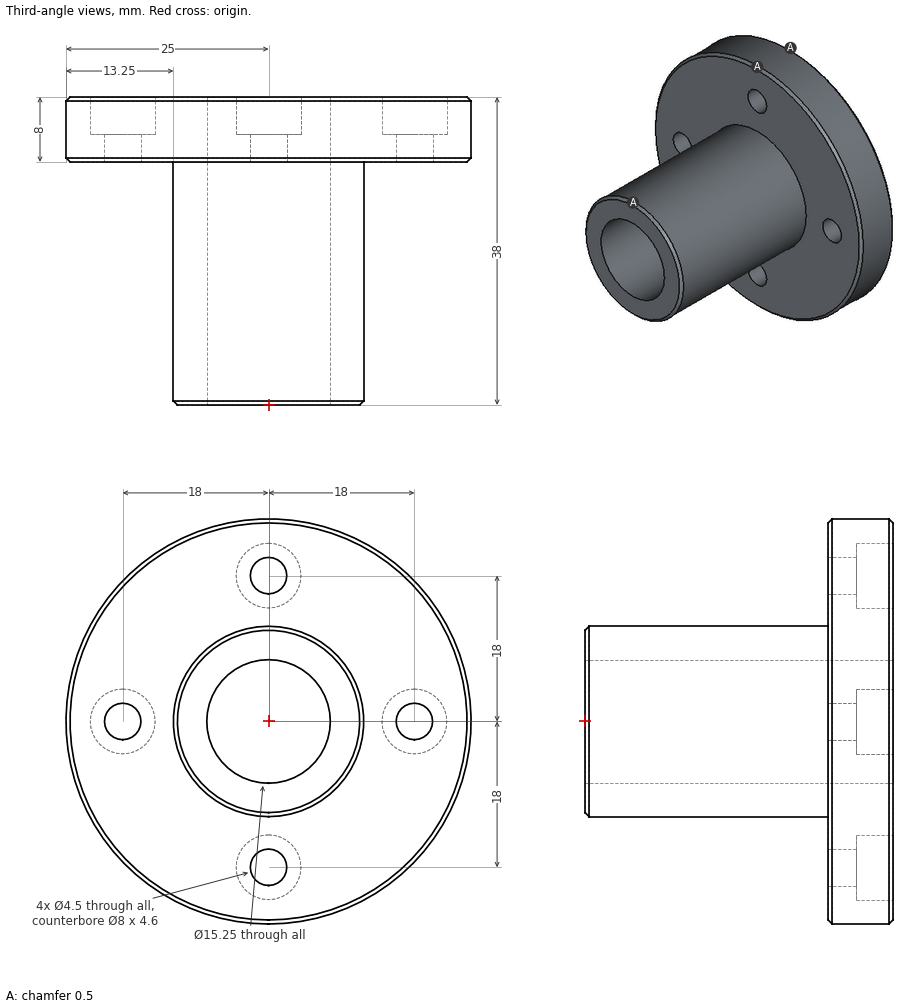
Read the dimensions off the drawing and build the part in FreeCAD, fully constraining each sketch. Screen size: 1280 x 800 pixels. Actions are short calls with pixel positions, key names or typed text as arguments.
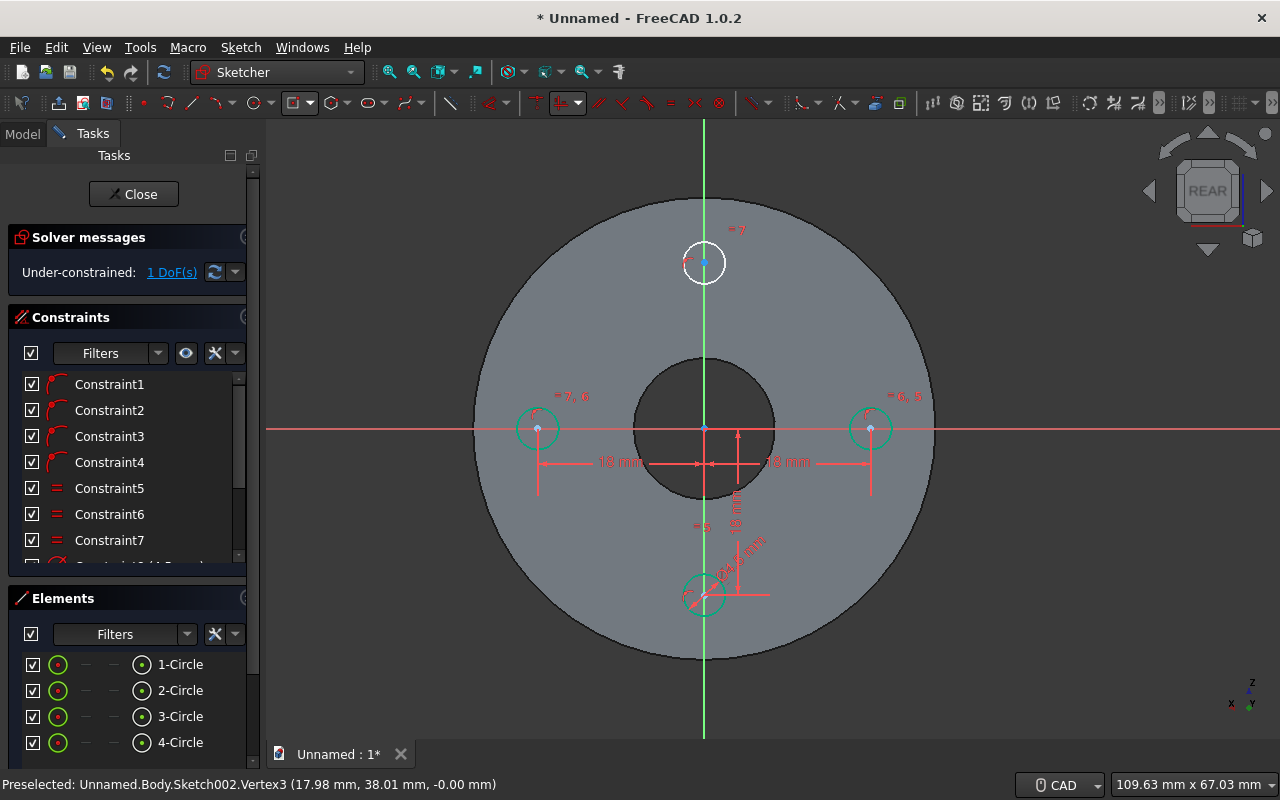
click(704, 263)
click(738, 346)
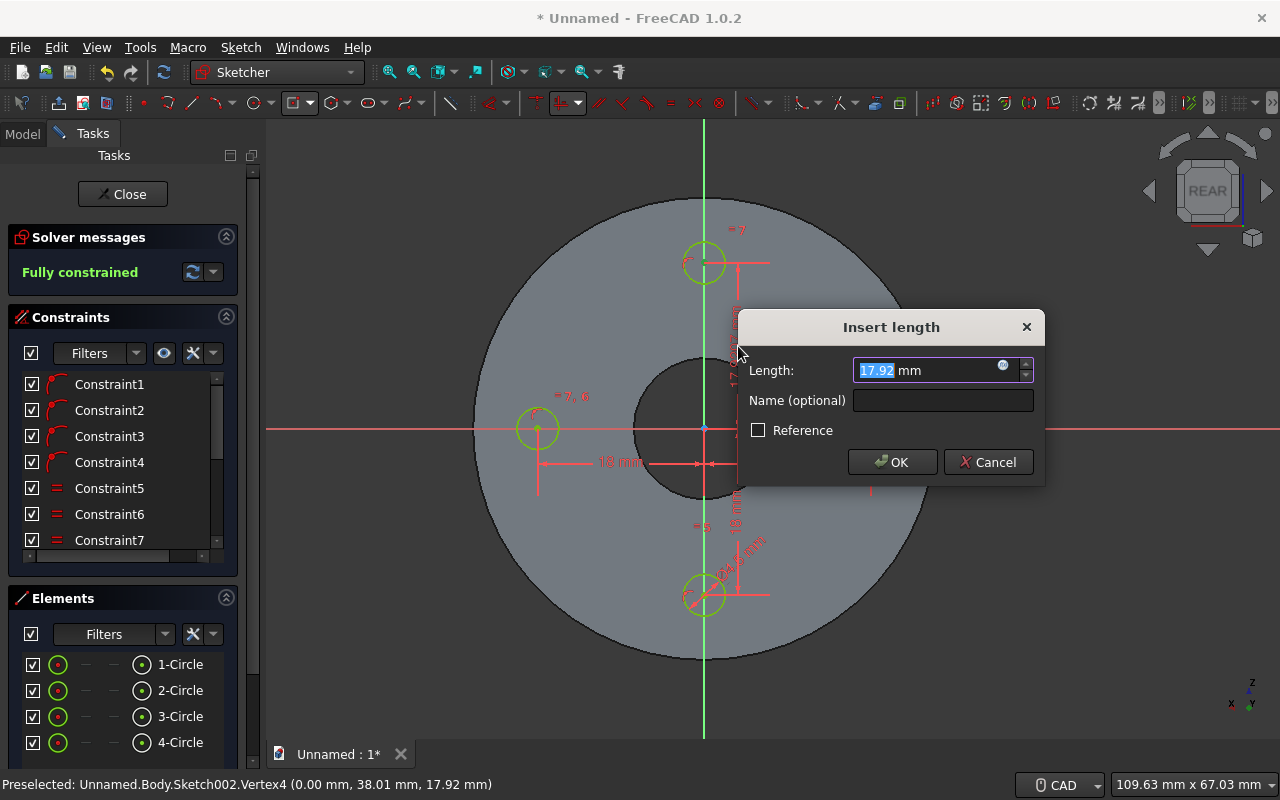
text(18)
key(Return)
key(Escape)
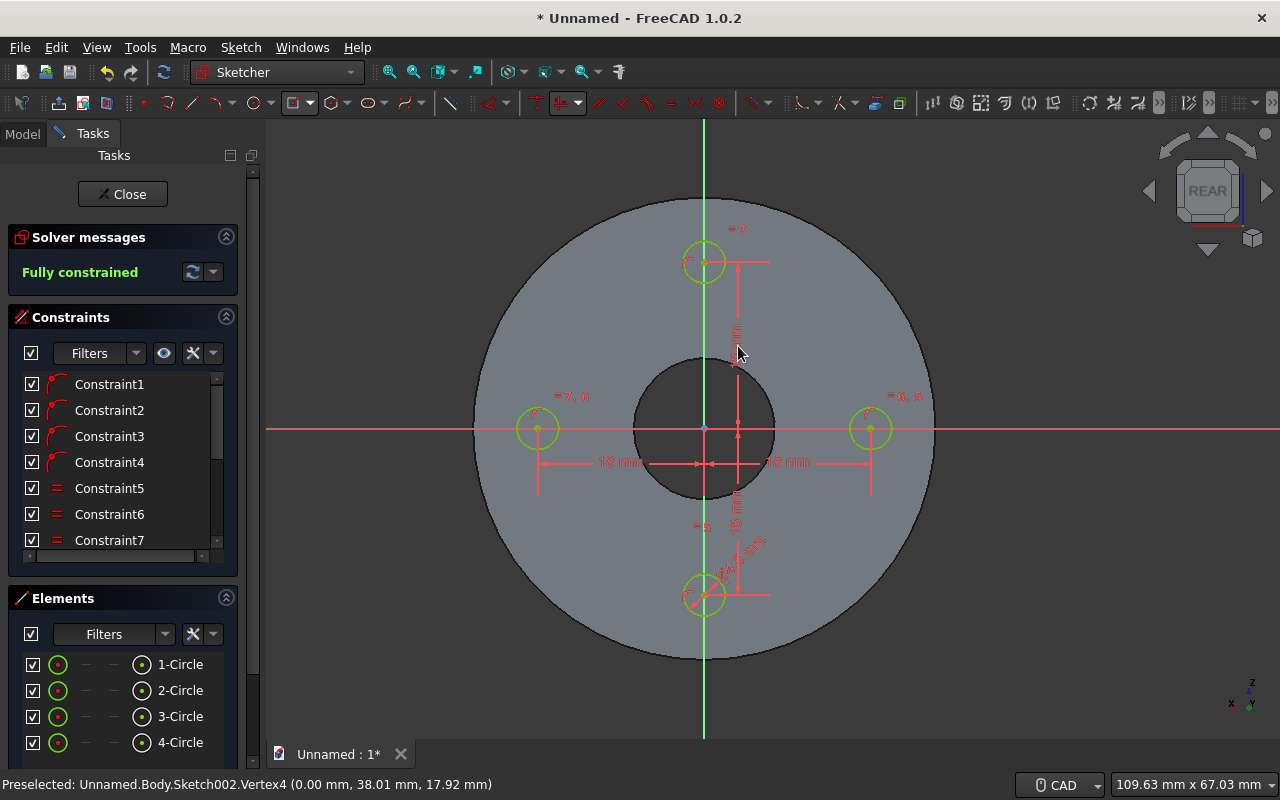
click(123, 194)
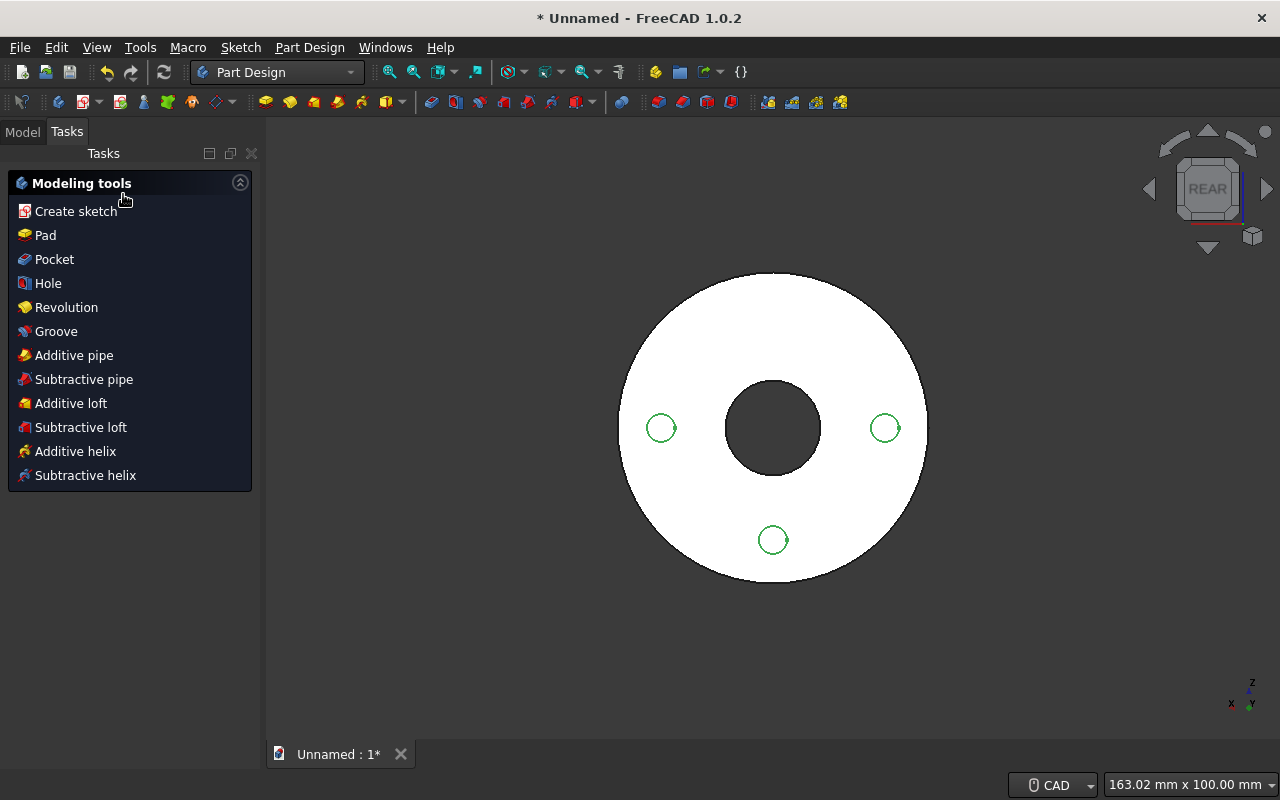
click(456, 102)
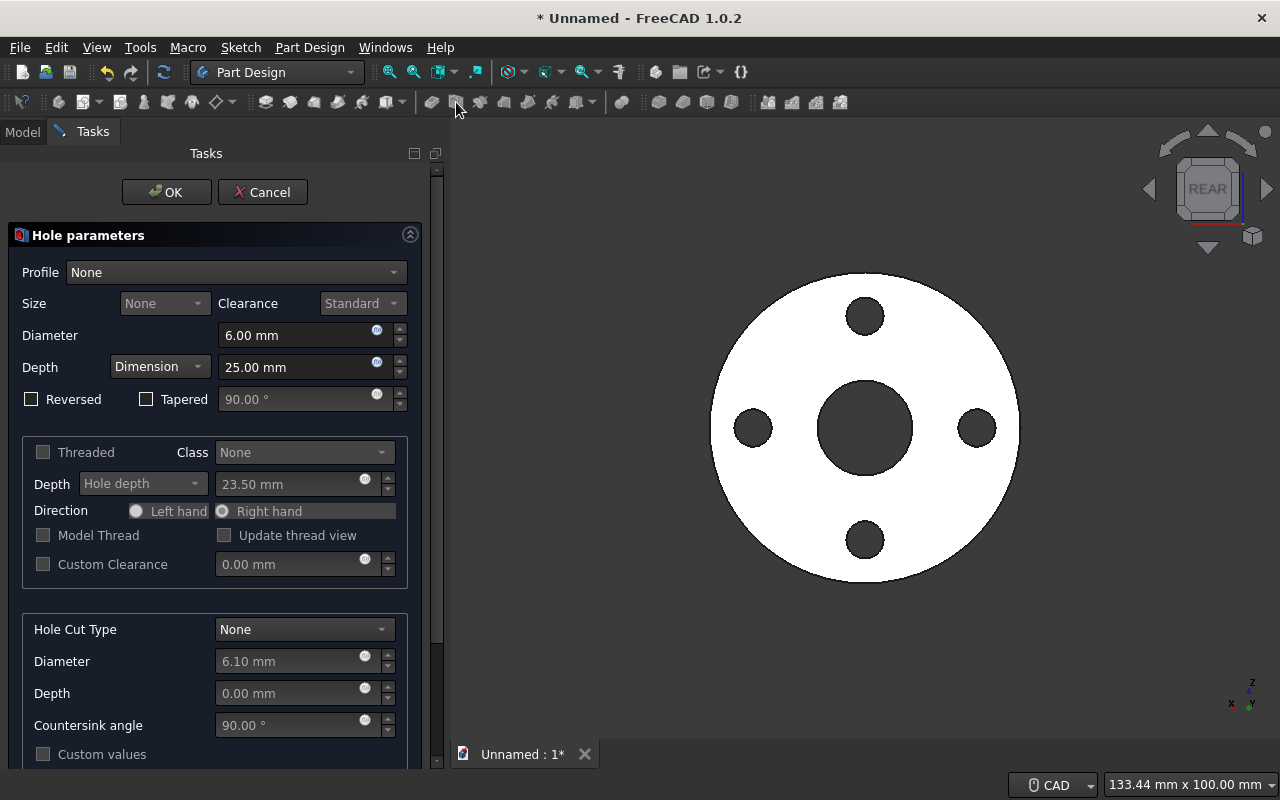
triple_click(305, 335)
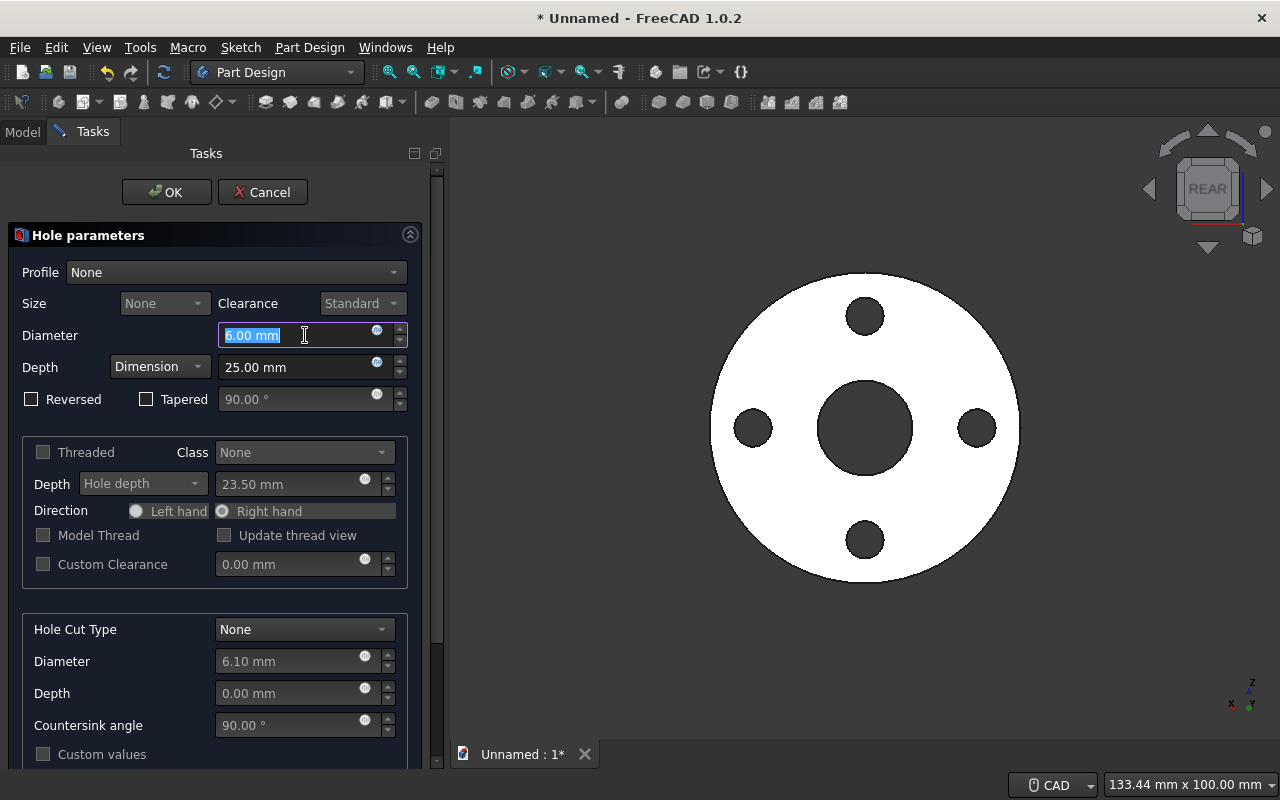
text(4.5)
key(Tab)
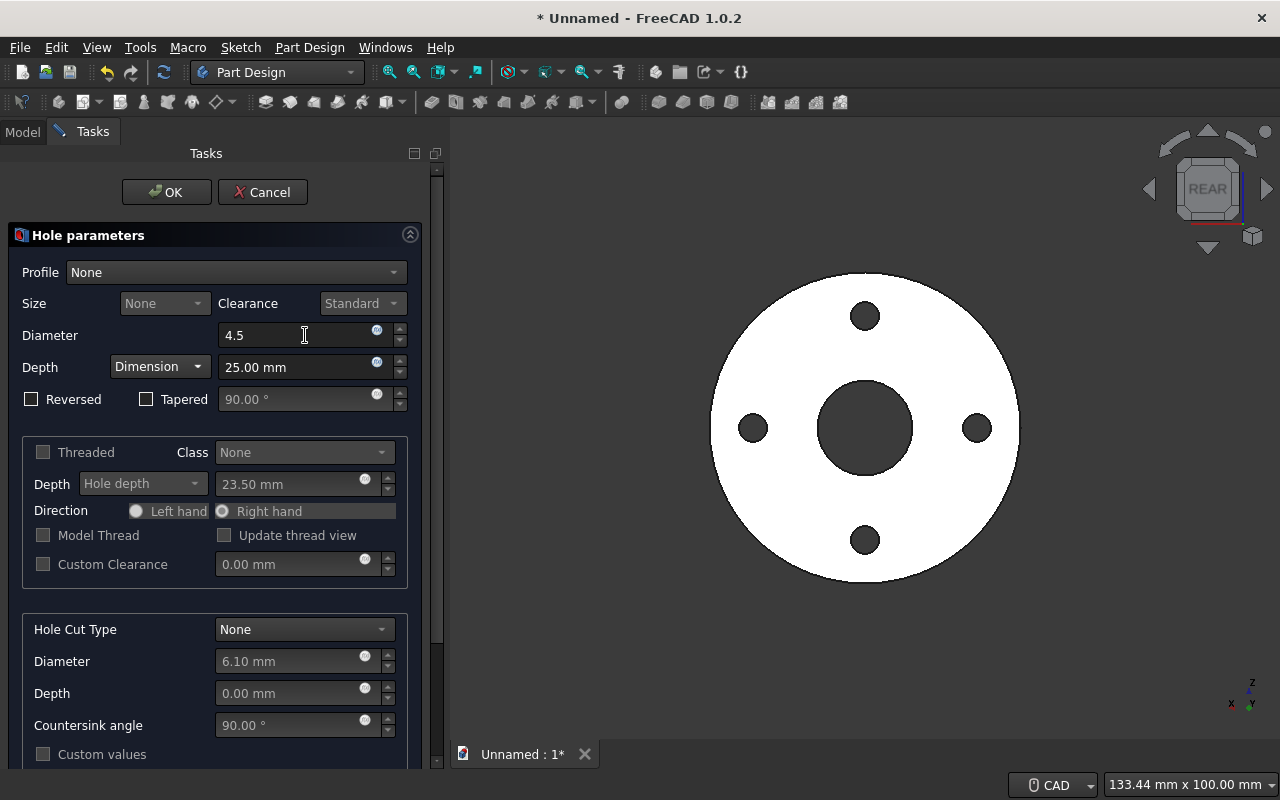
click(161, 366)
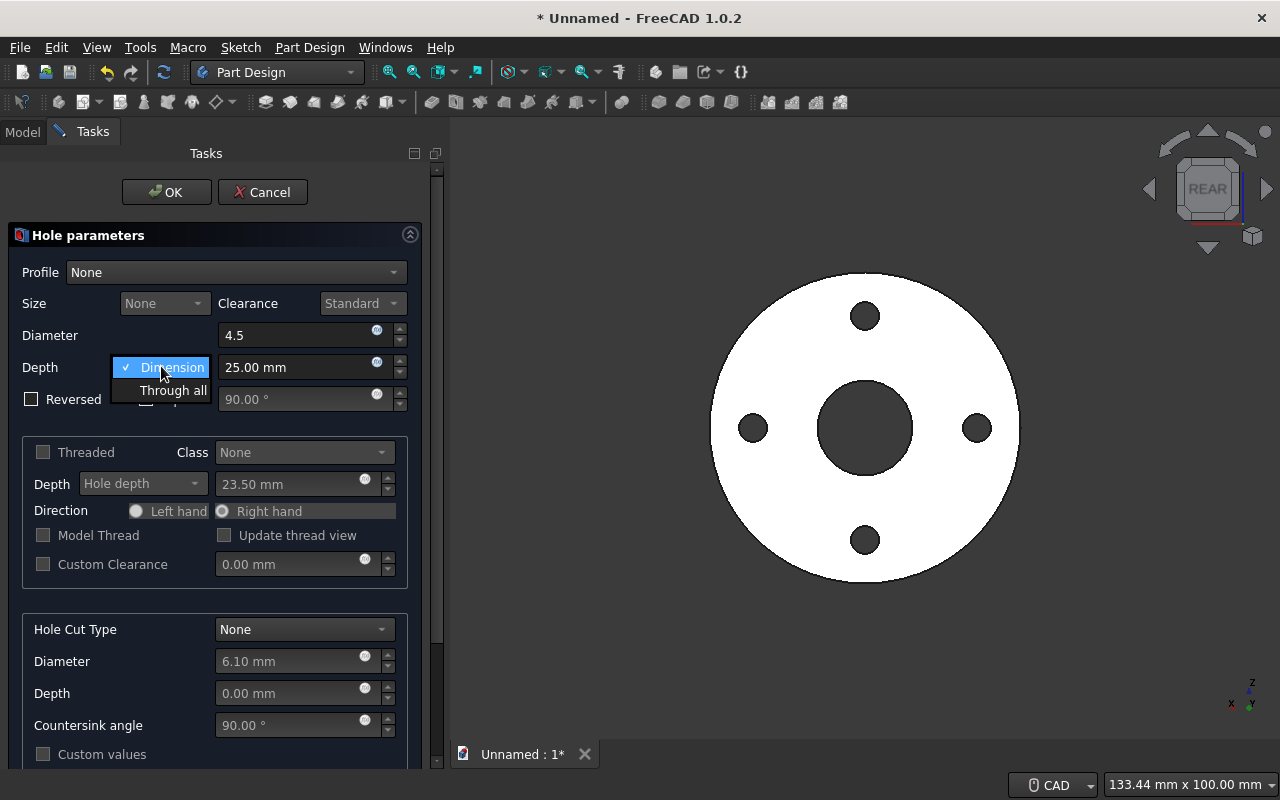
click(160, 390)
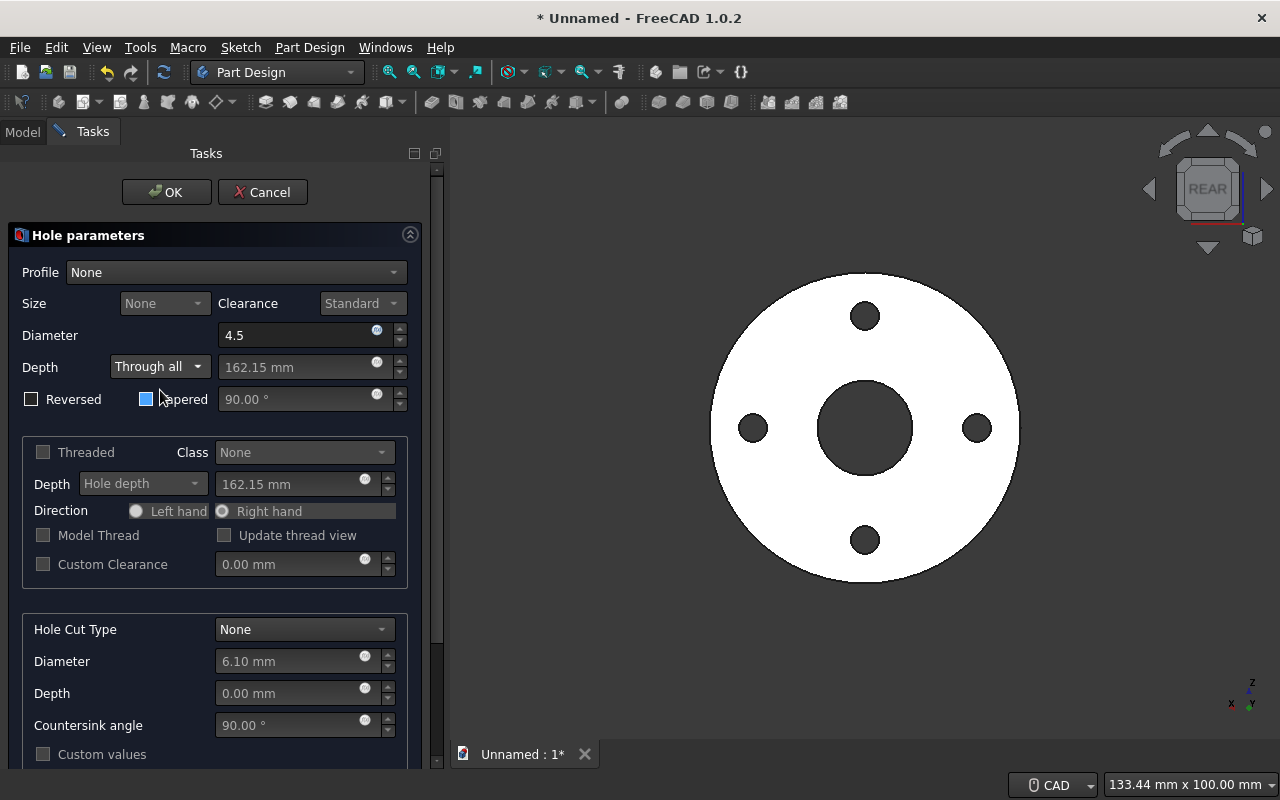
click(306, 630)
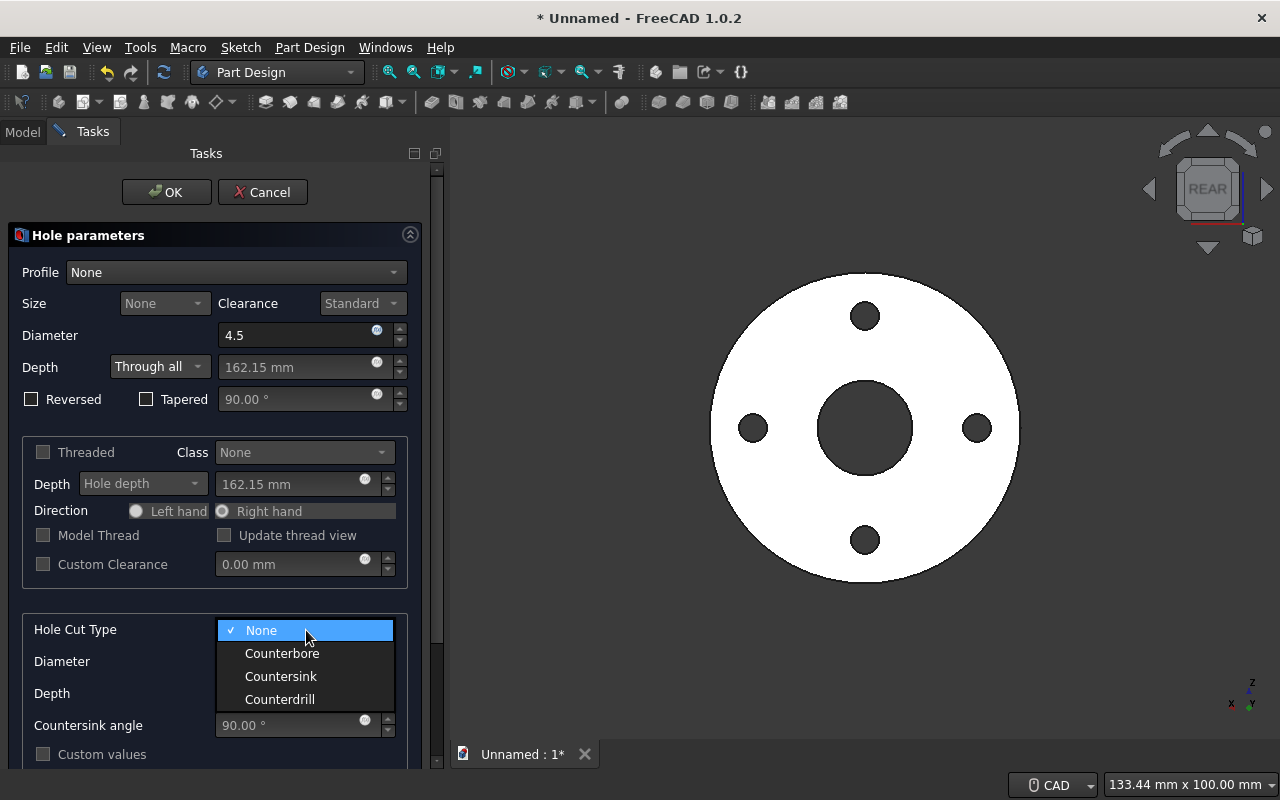
click(304, 654)